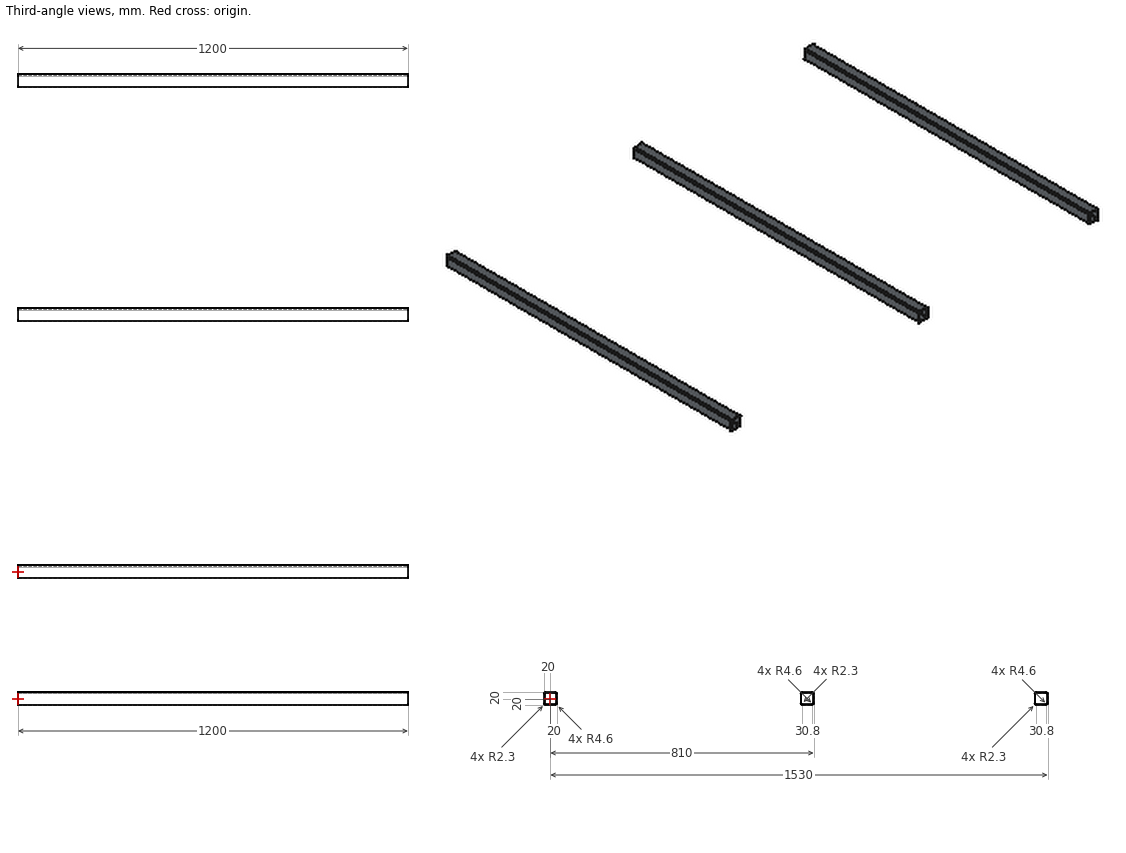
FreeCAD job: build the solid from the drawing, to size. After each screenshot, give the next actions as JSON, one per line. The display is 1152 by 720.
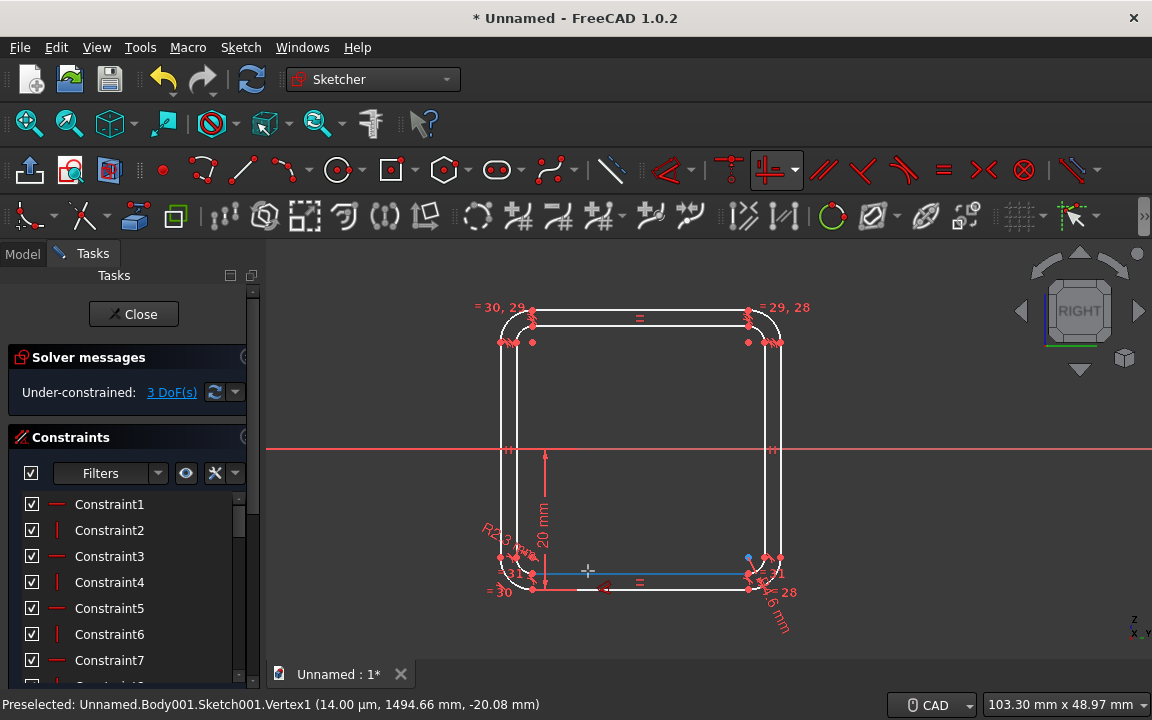
{"action": "left_click", "coordinate": [748, 310]}
{"action": "left_click", "coordinate": [806, 380]}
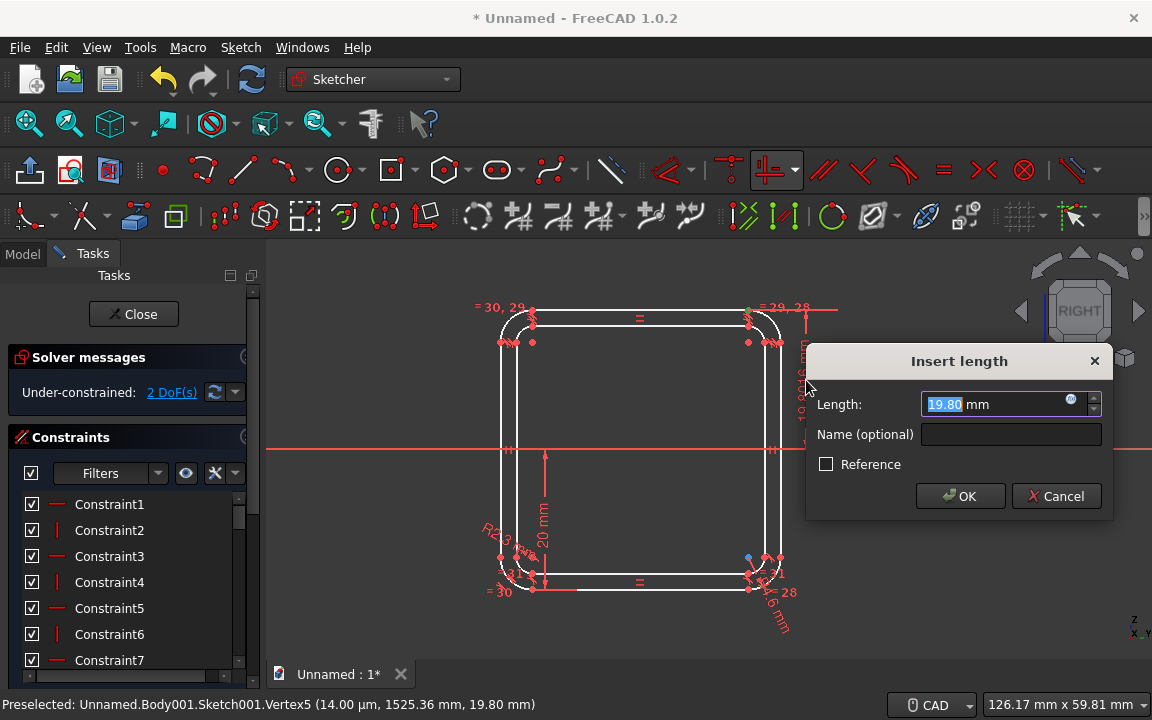
{"action": "type", "text": "20"}
{"action": "key", "text": "Return"}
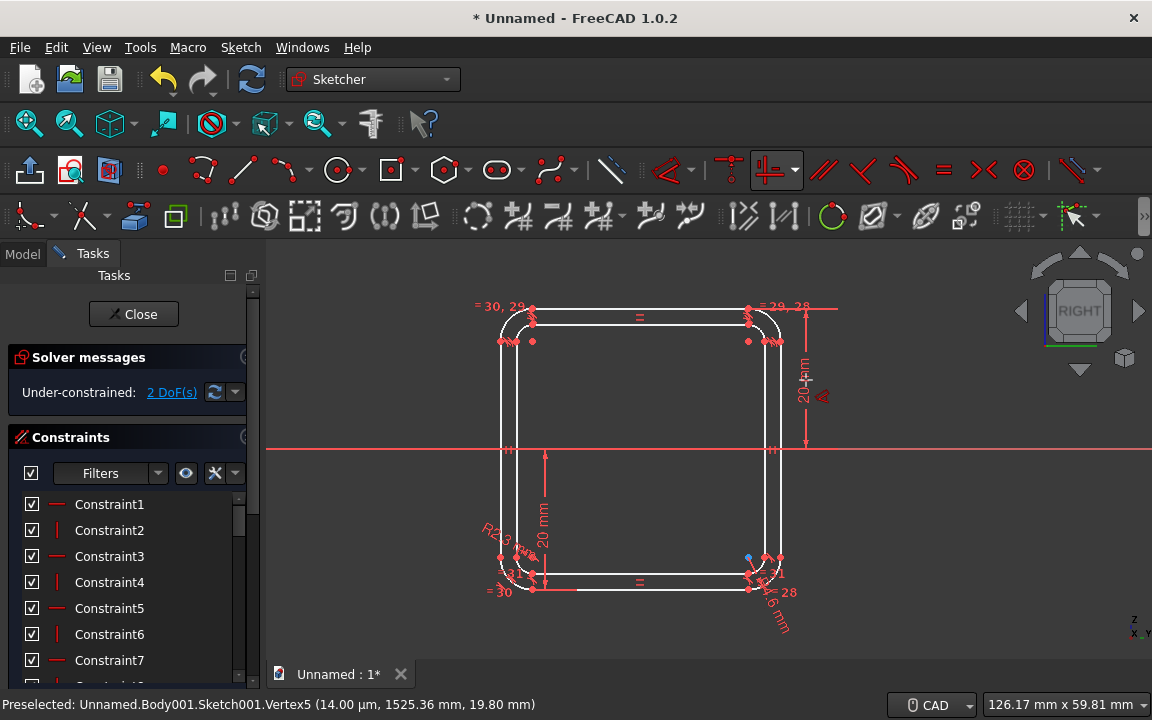
{"action": "left_click", "coordinate": [597, 590]}
{"action": "left_click", "coordinate": [641, 624]}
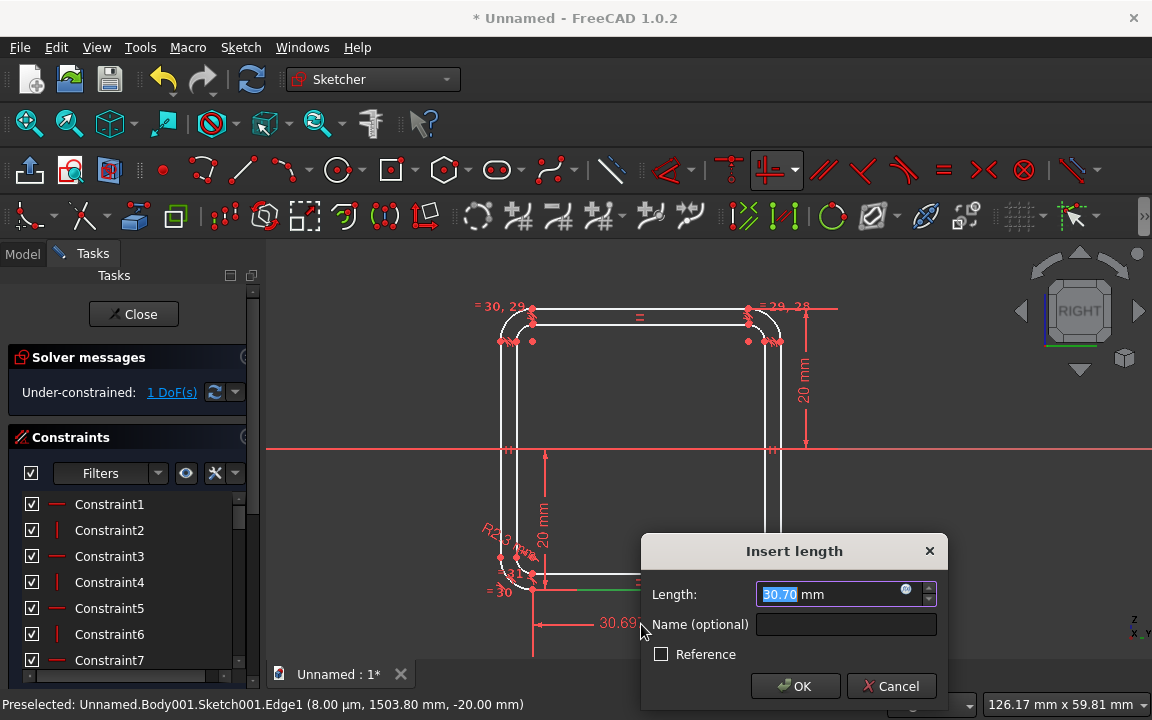
{"action": "type", "text": "30.8"}
{"action": "key", "text": "Return"}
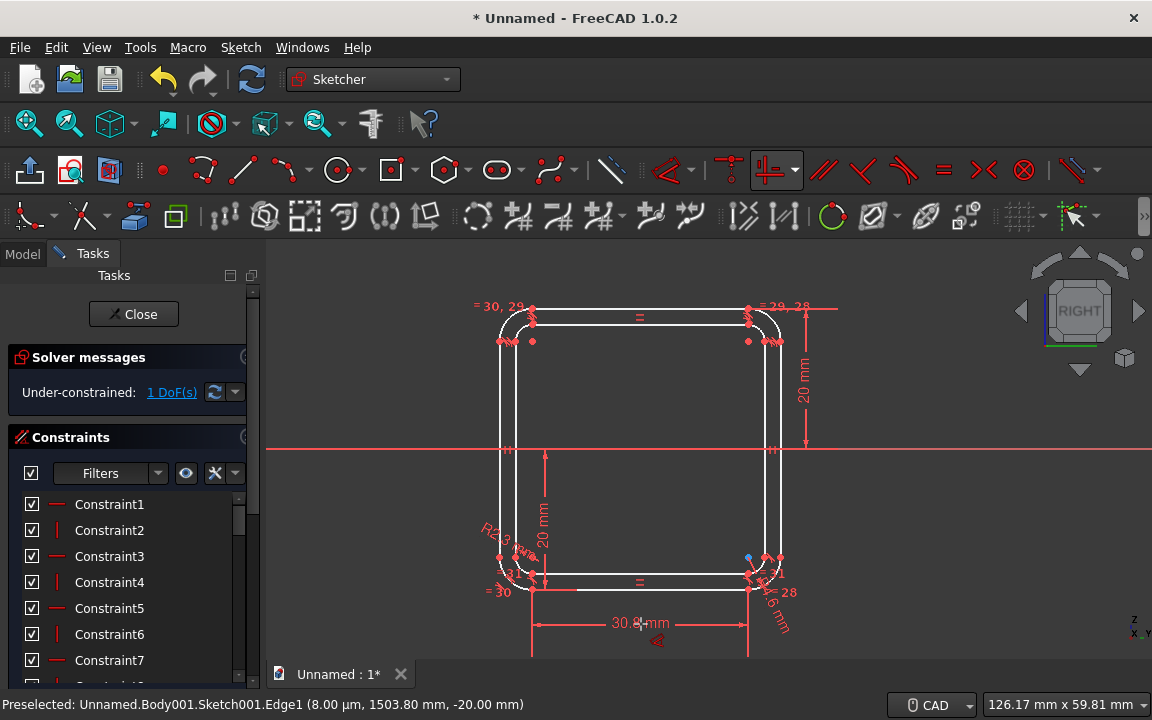
{"action": "left_click", "coordinate": [781, 557]}
{"action": "left_click", "coordinate": [425, 591]}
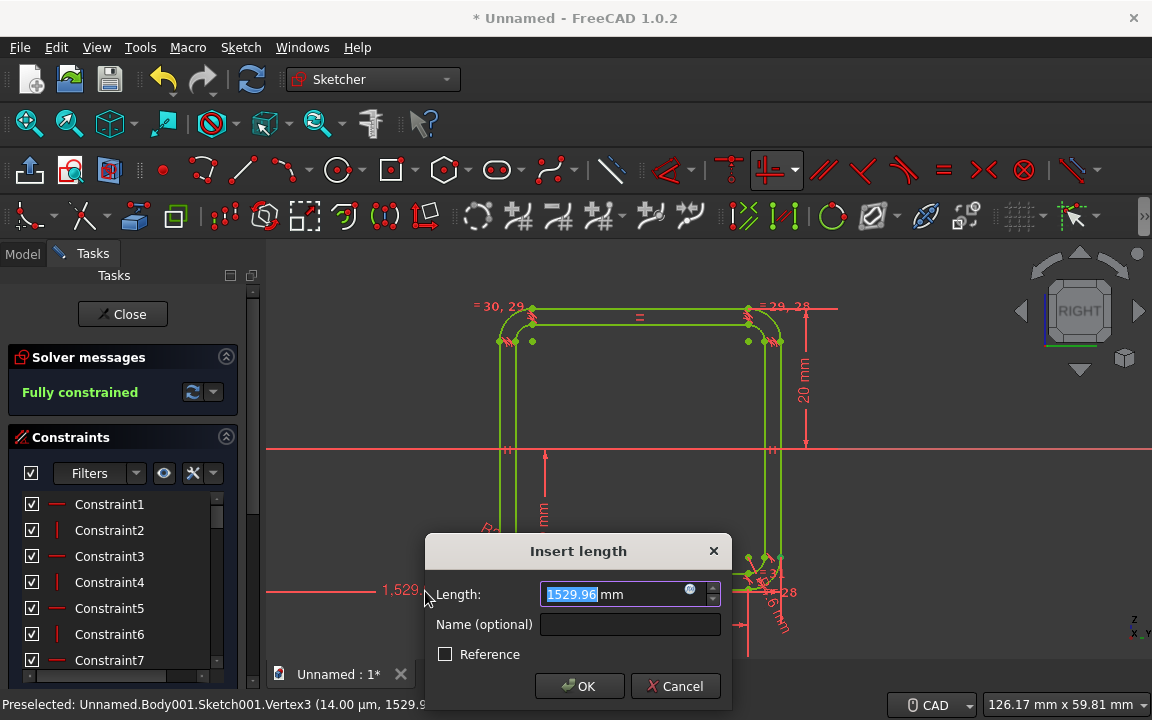
{"action": "type", "text": "1530"}
{"action": "key", "text": "Return"}
{"action": "key", "text": "Escape"}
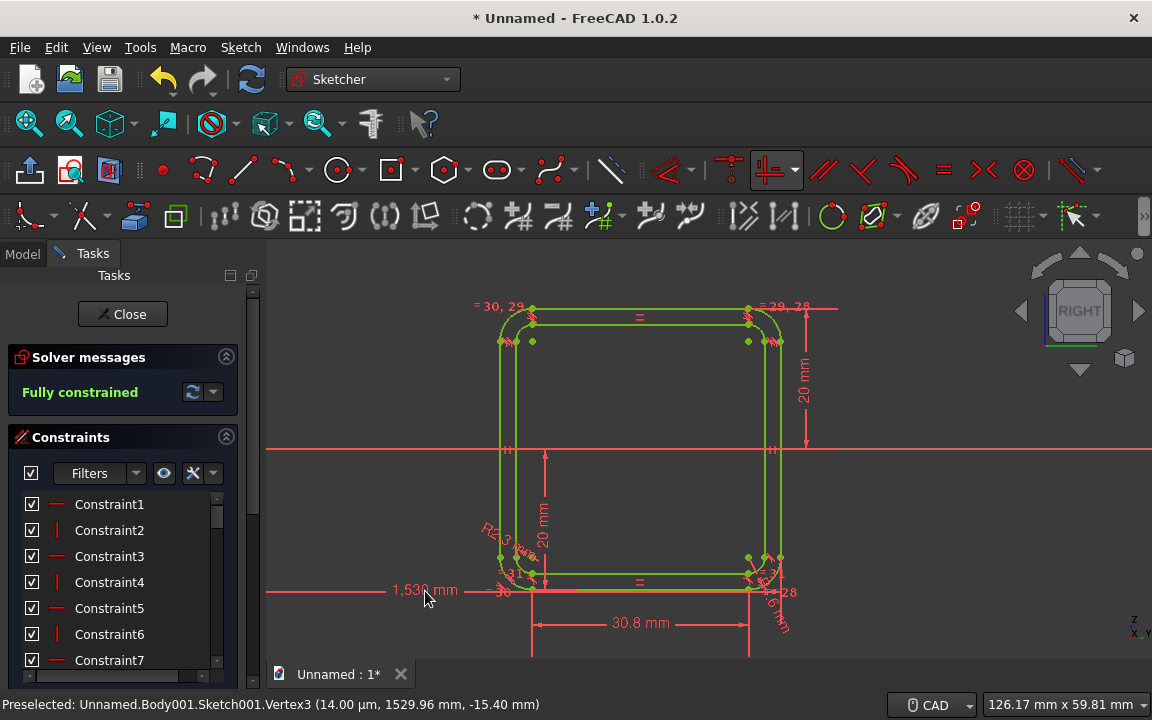
{"action": "left_click", "coordinate": [123, 314]}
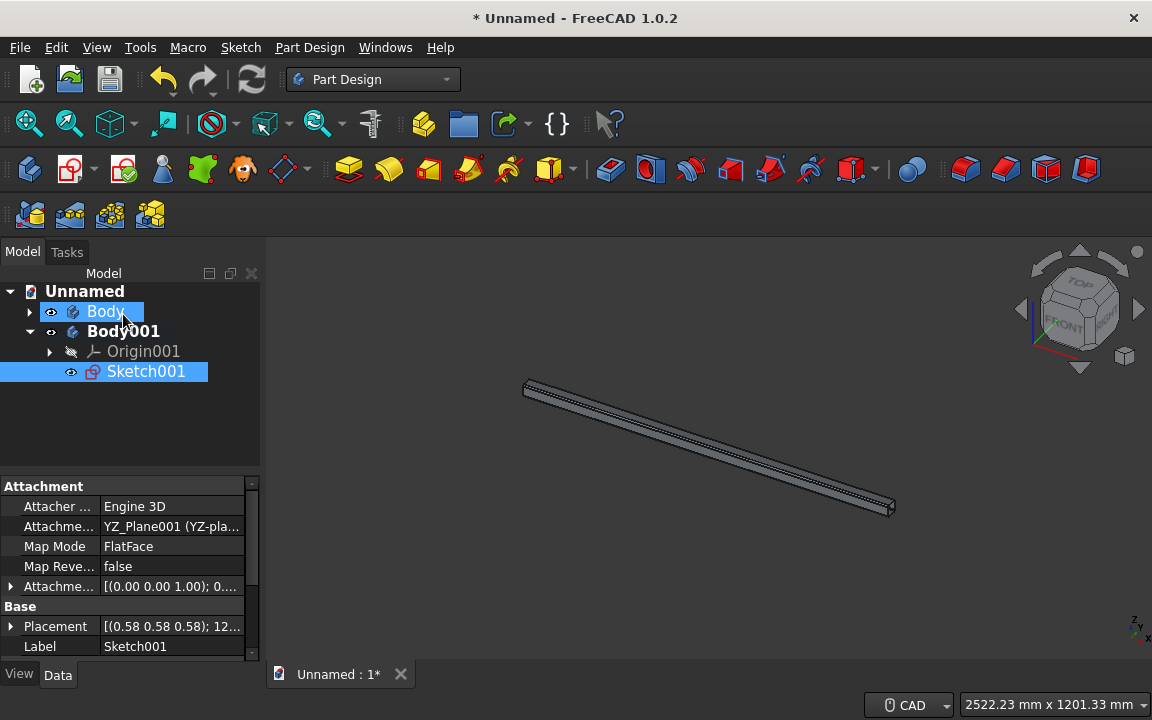
{"action": "left_click", "coordinate": [350, 170]}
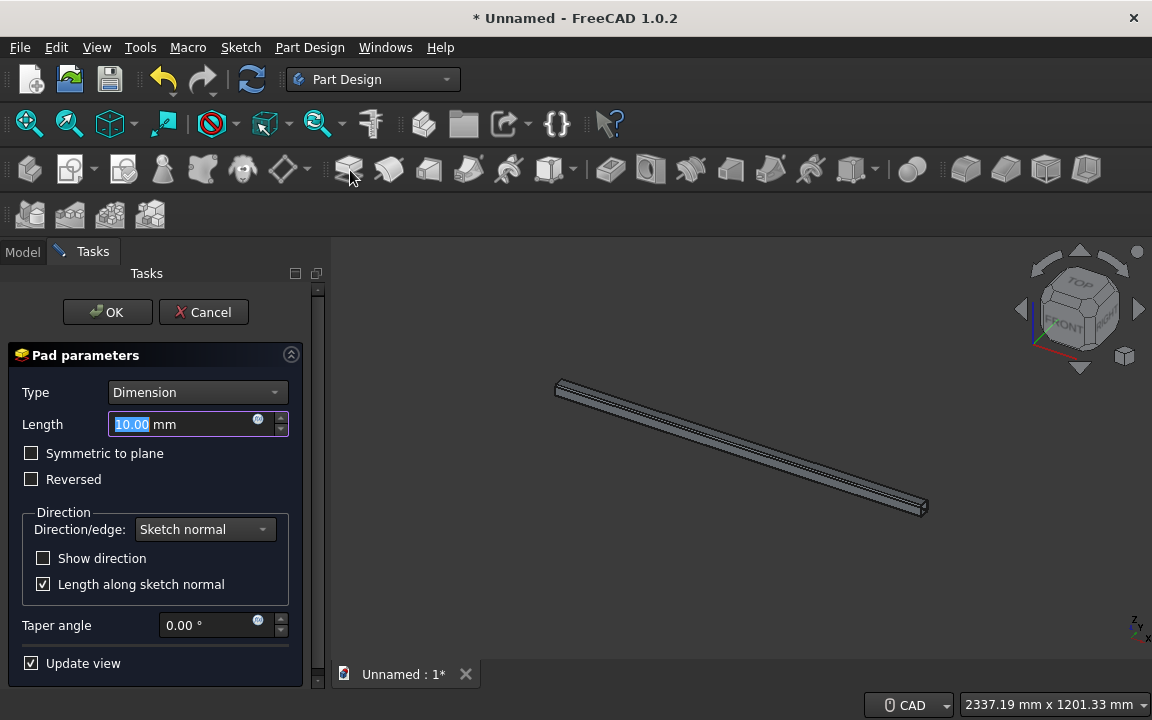
{"action": "type", "text": "1200"}
{"action": "key", "text": "Tab"}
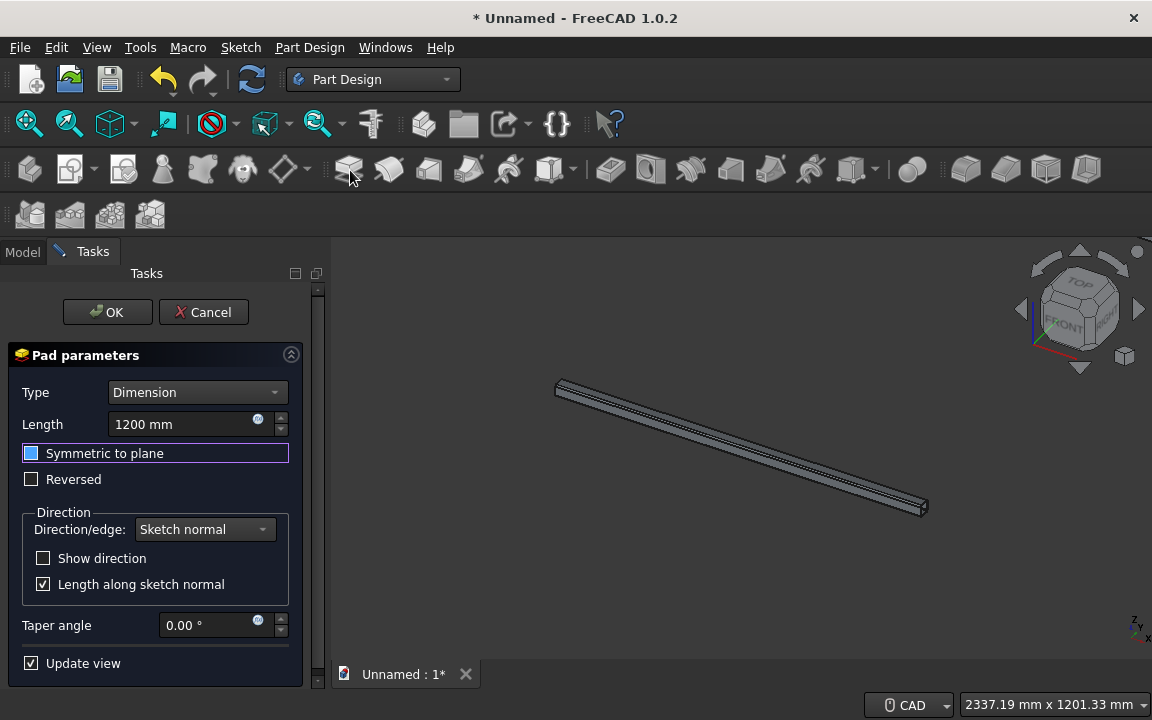
{"action": "left_click", "coordinate": [108, 312]}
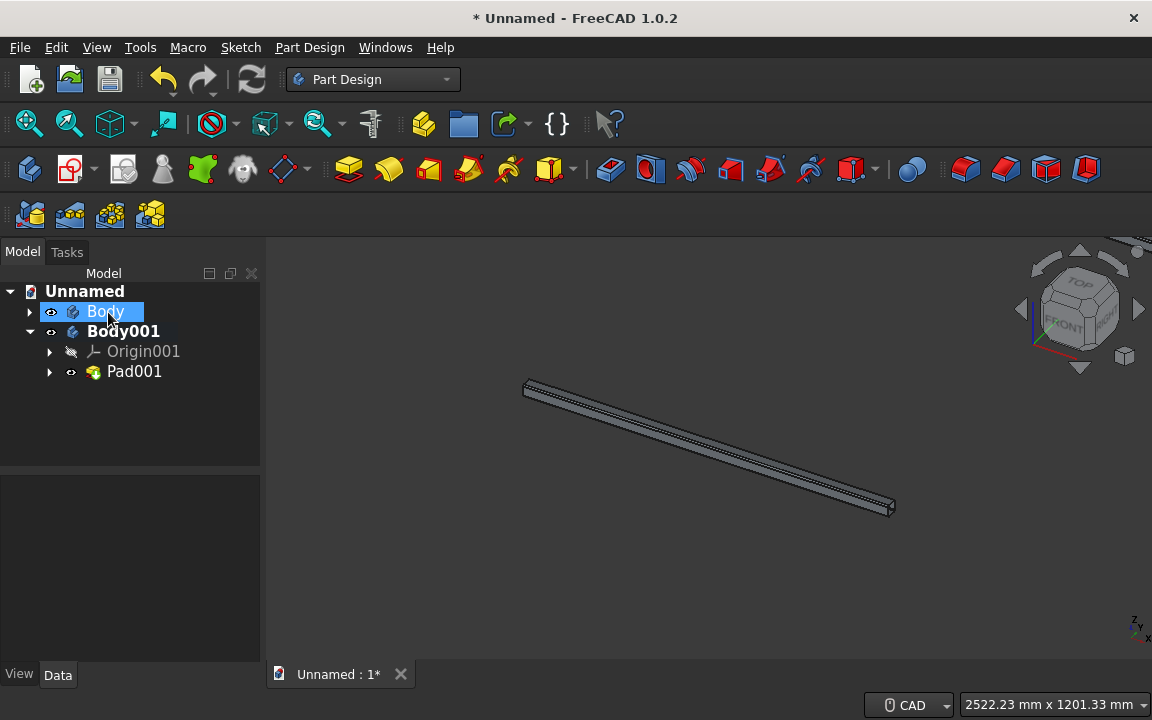
{"action": "left_click", "coordinate": [30, 124]}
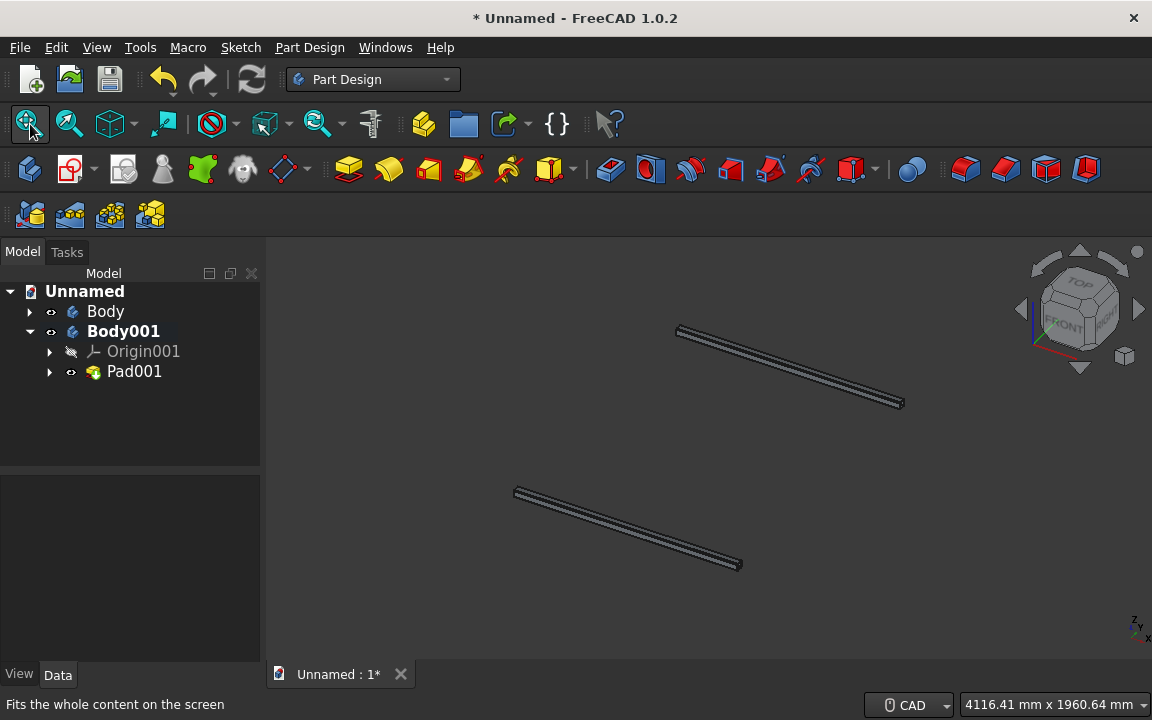
{"action": "left_click", "coordinate": [30, 170]}